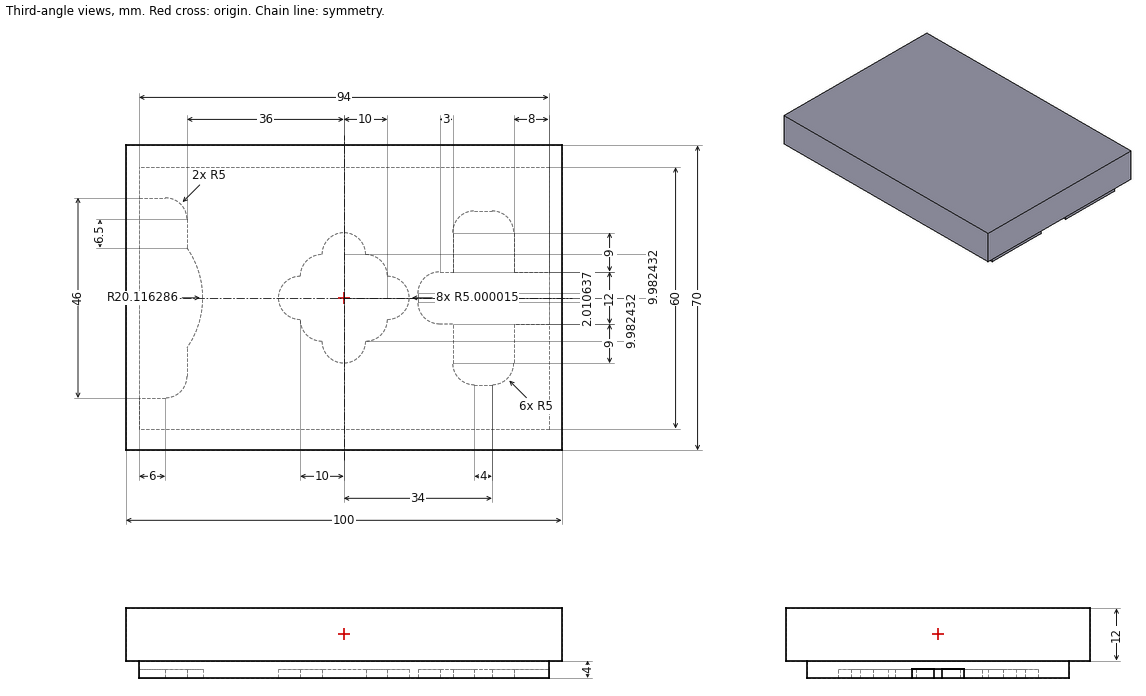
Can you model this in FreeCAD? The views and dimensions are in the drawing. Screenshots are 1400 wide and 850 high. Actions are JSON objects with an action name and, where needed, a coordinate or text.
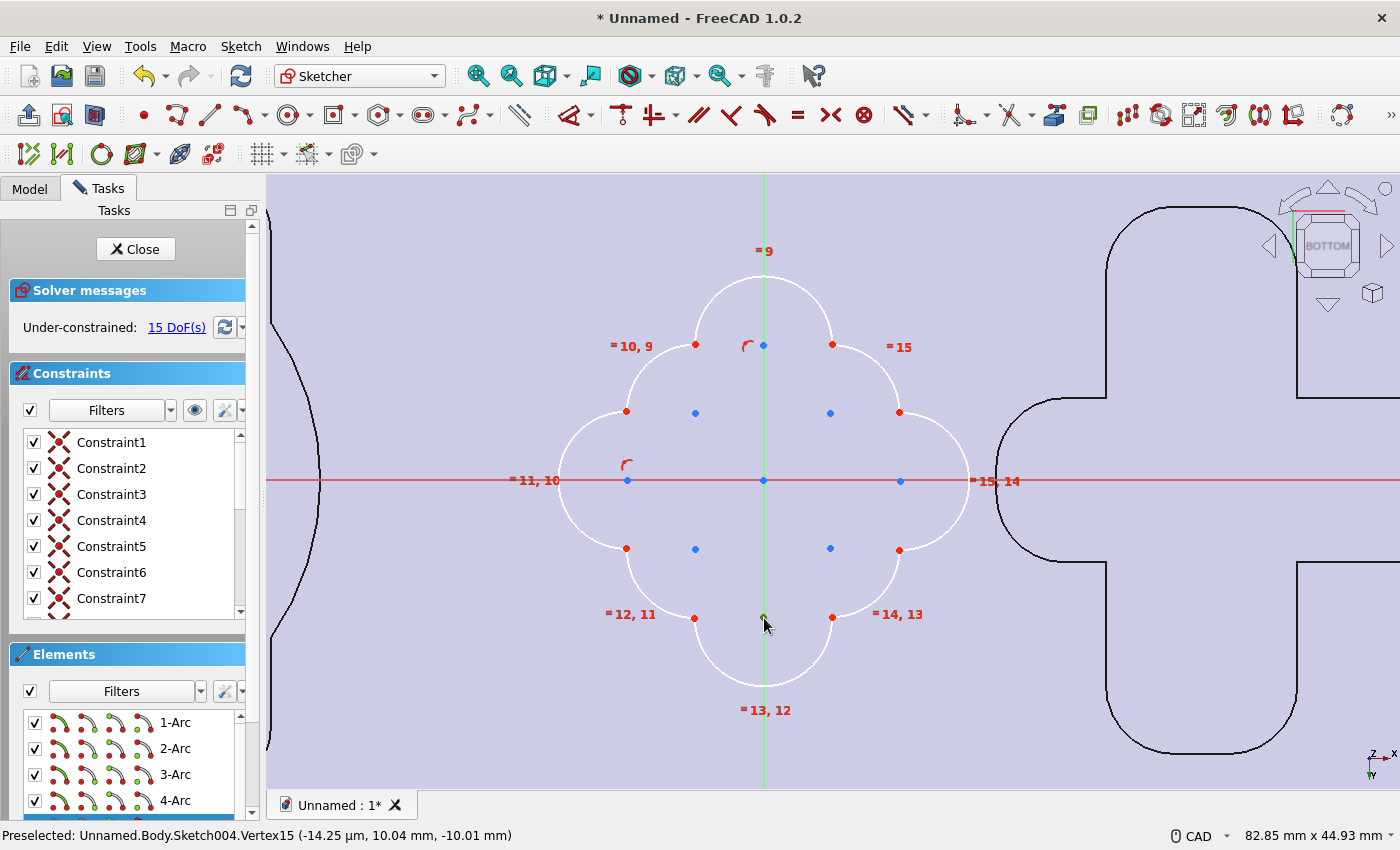
{"action": "left_click", "coordinate": [764, 721]}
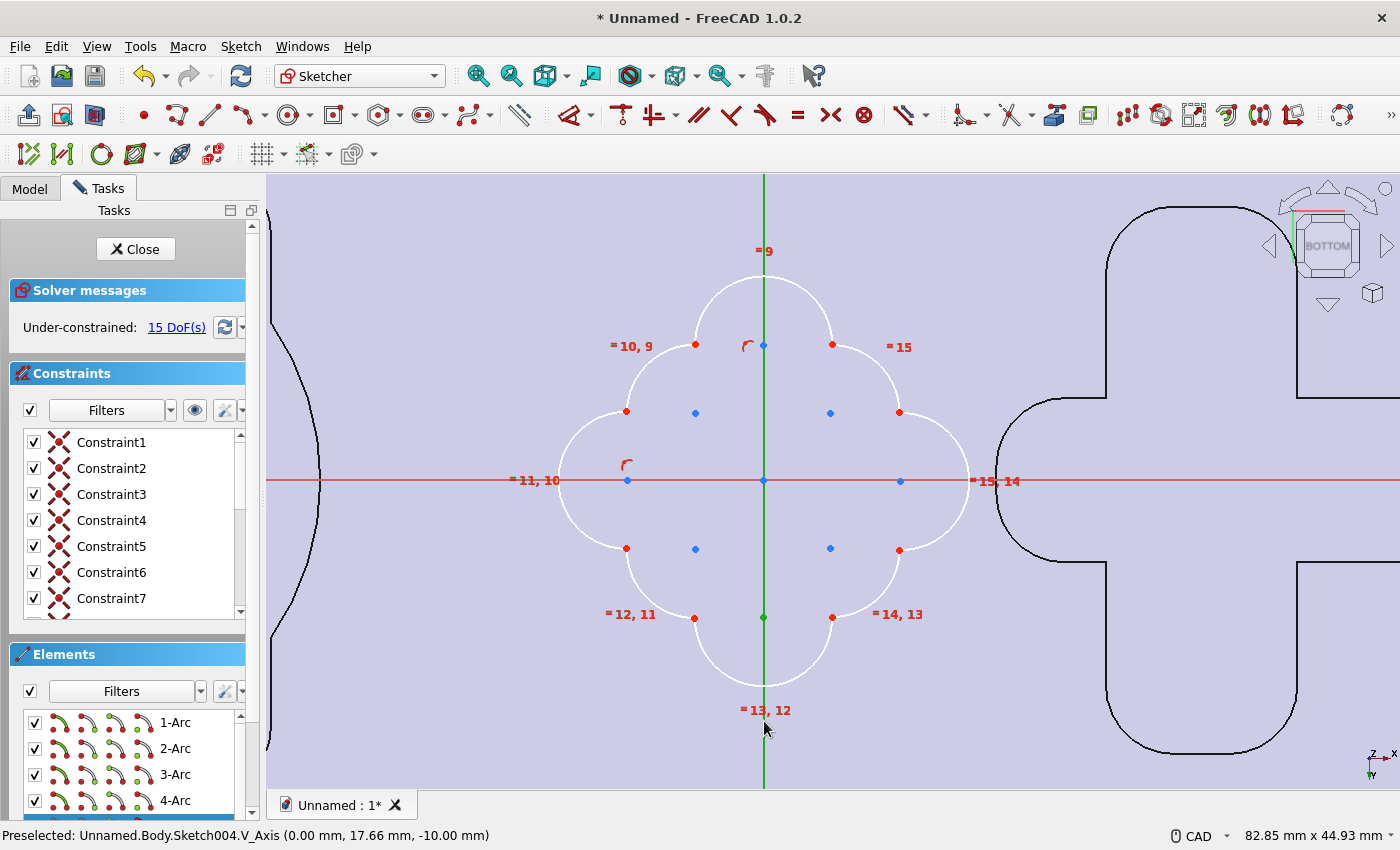
{"action": "left_click", "coordinate": [621, 116]}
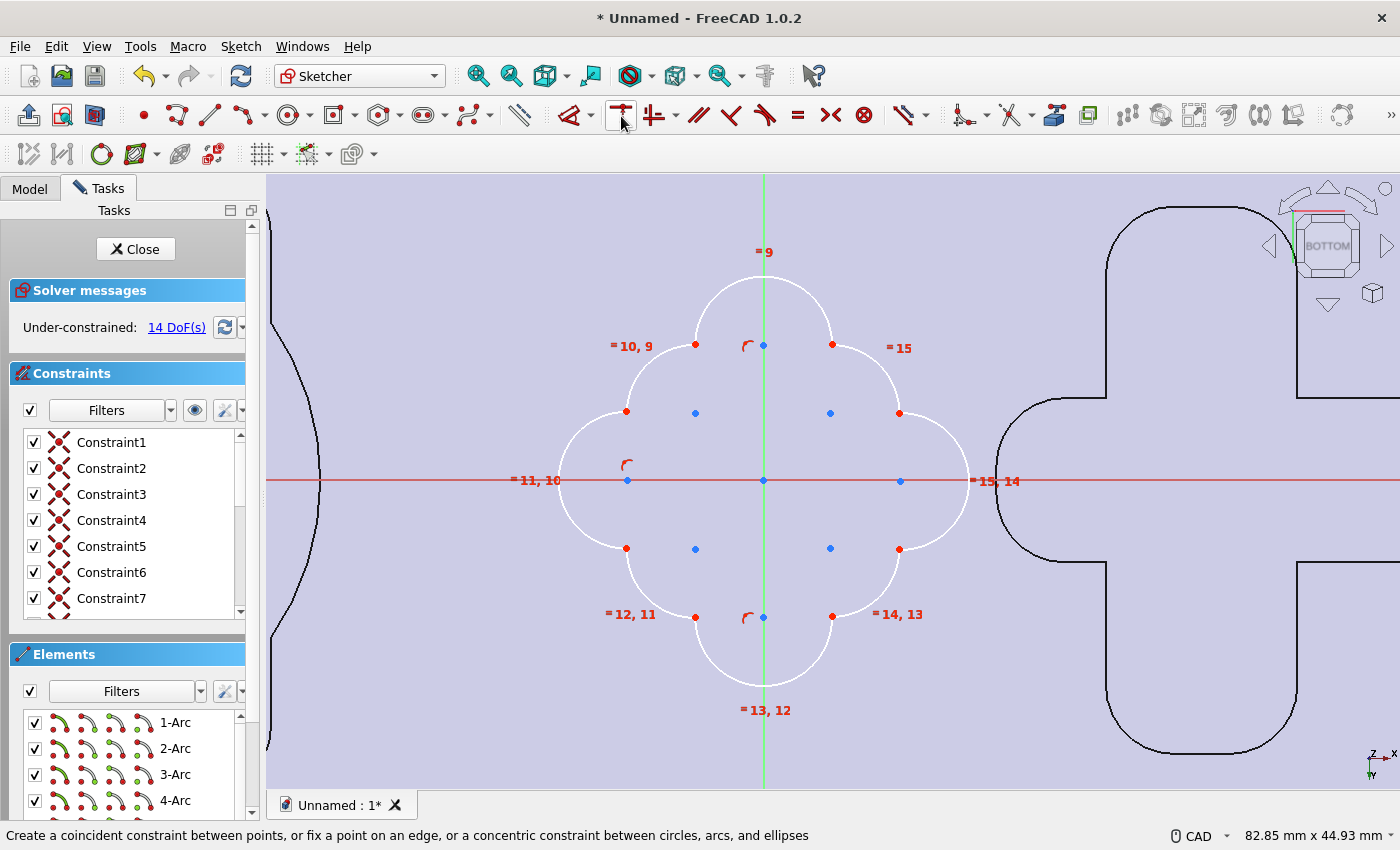
{"action": "left_click", "coordinate": [901, 482]}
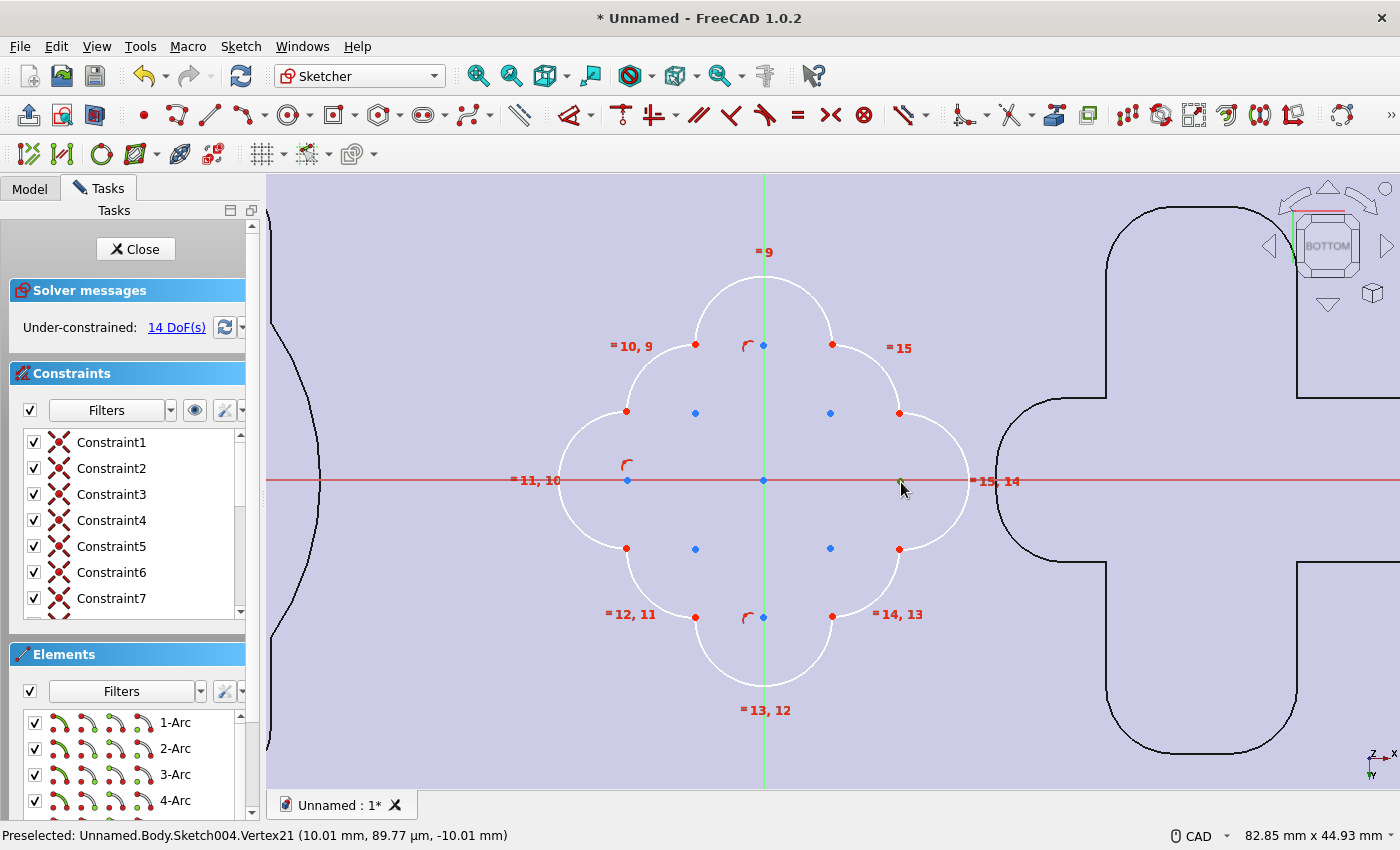
{"action": "left_click", "coordinate": [361, 480]}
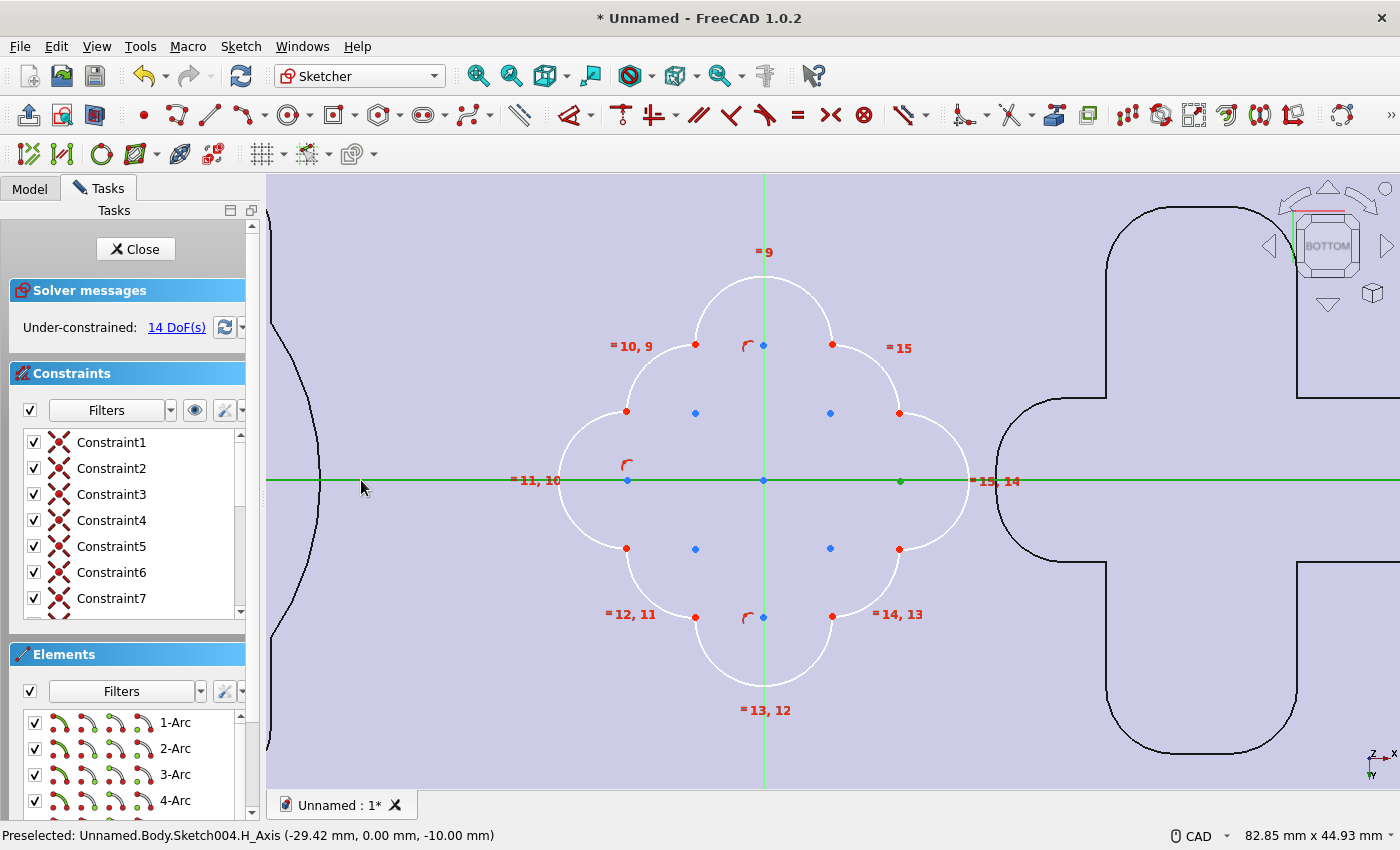
{"action": "left_click", "coordinate": [621, 116]}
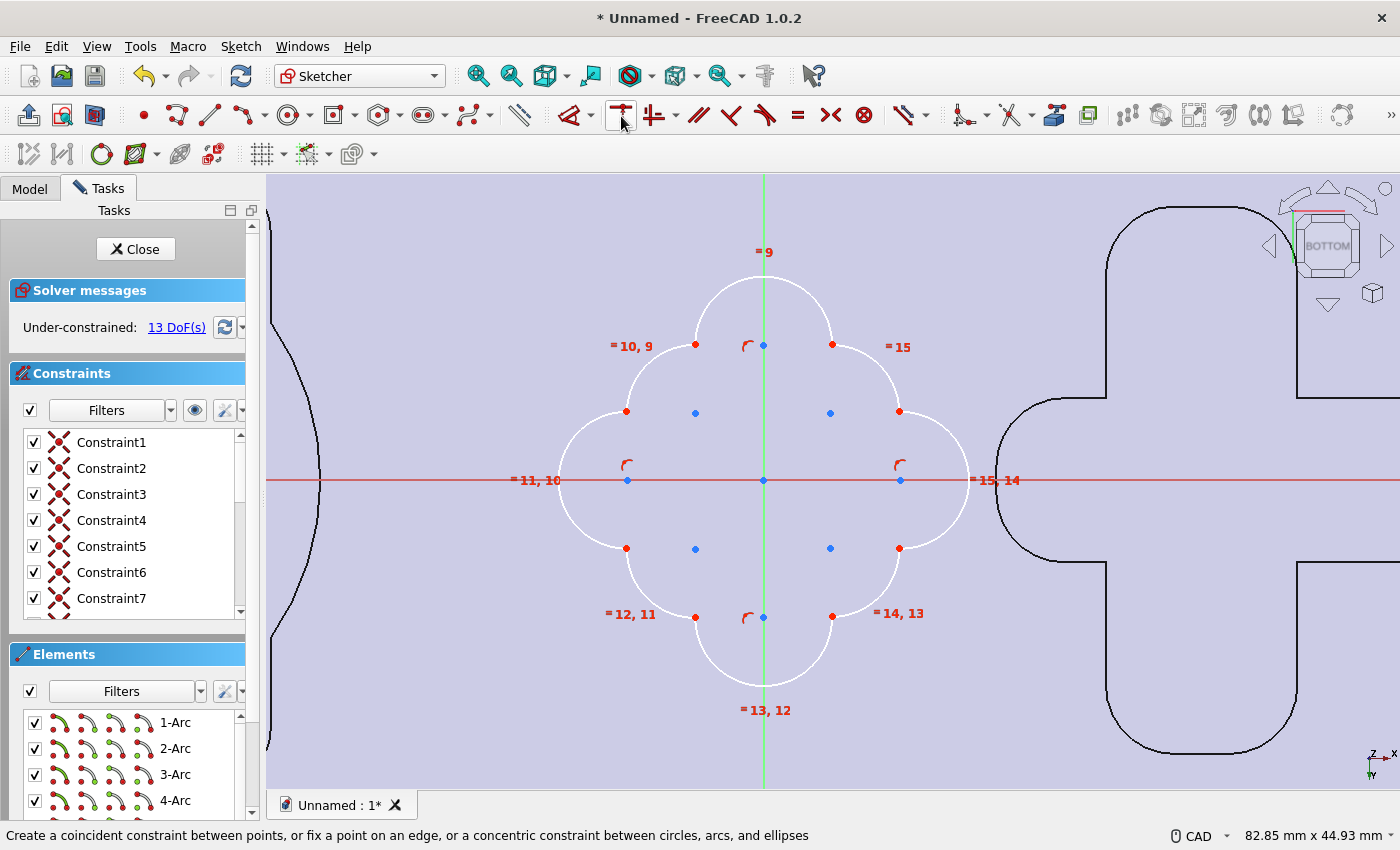
{"action": "left_click", "coordinate": [695, 413]}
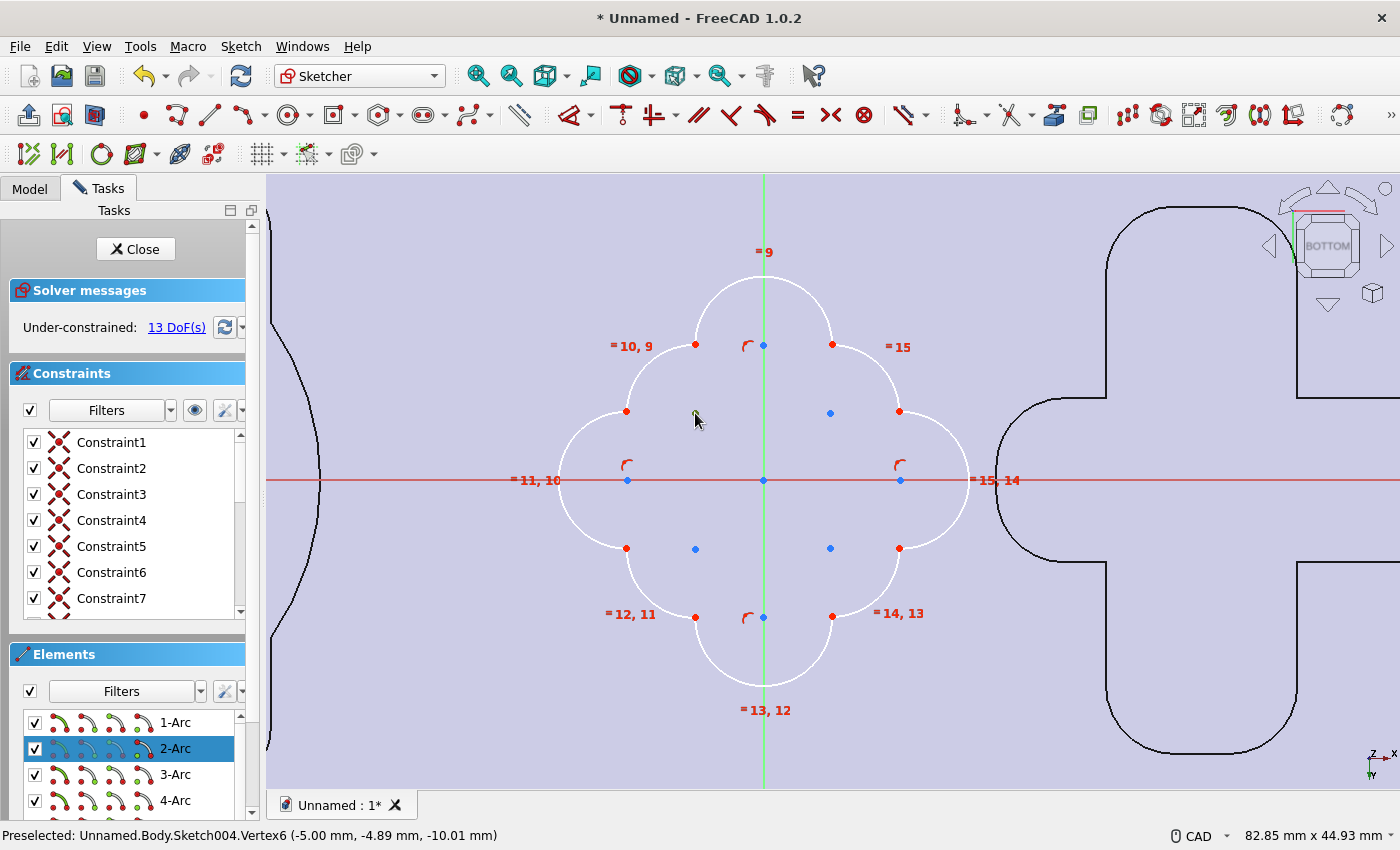
{"action": "left_click", "coordinate": [695, 549]}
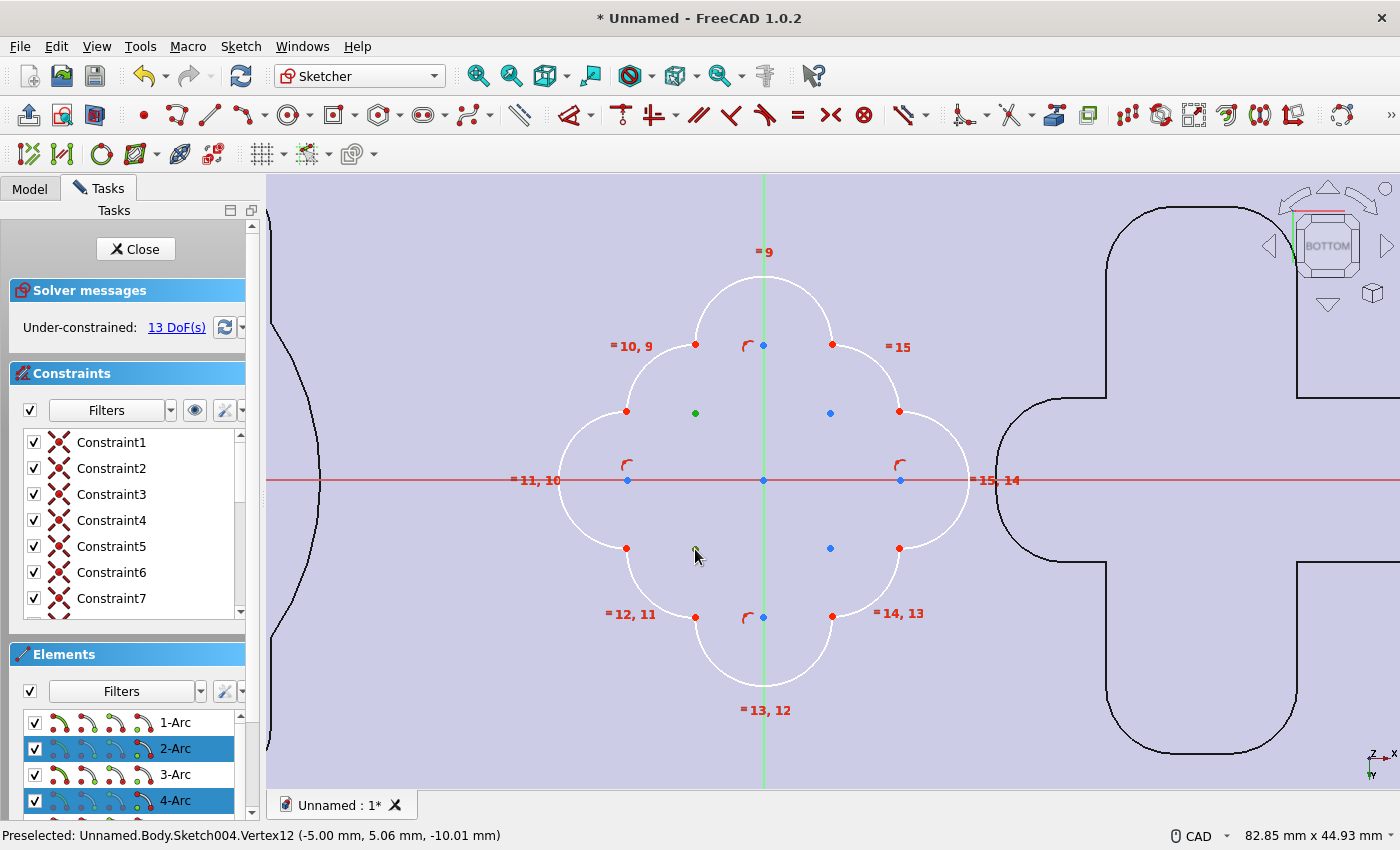
{"action": "left_click", "coordinate": [361, 480]}